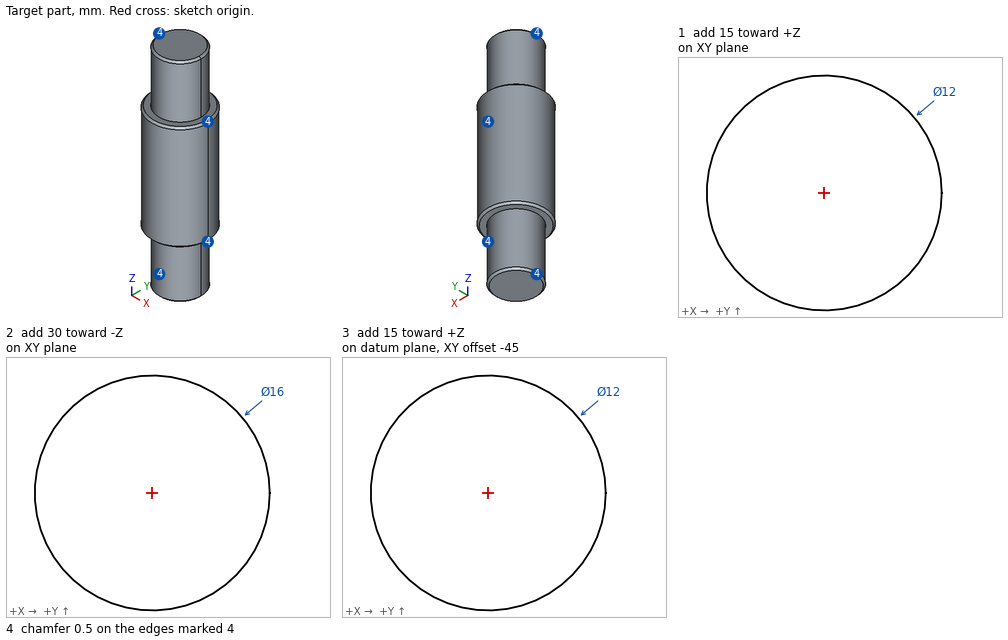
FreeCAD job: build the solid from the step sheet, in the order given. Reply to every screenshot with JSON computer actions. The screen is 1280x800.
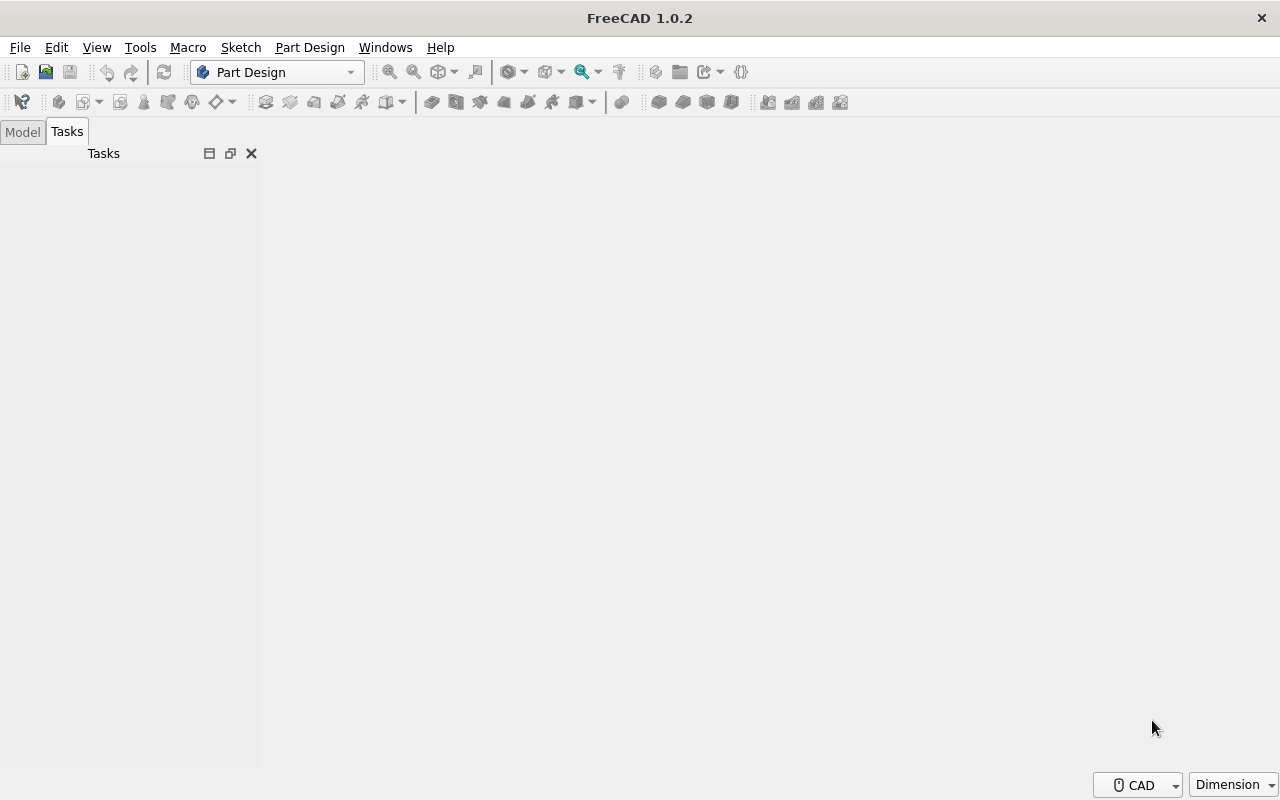
{"action": "left_click", "coordinate": [22, 72]}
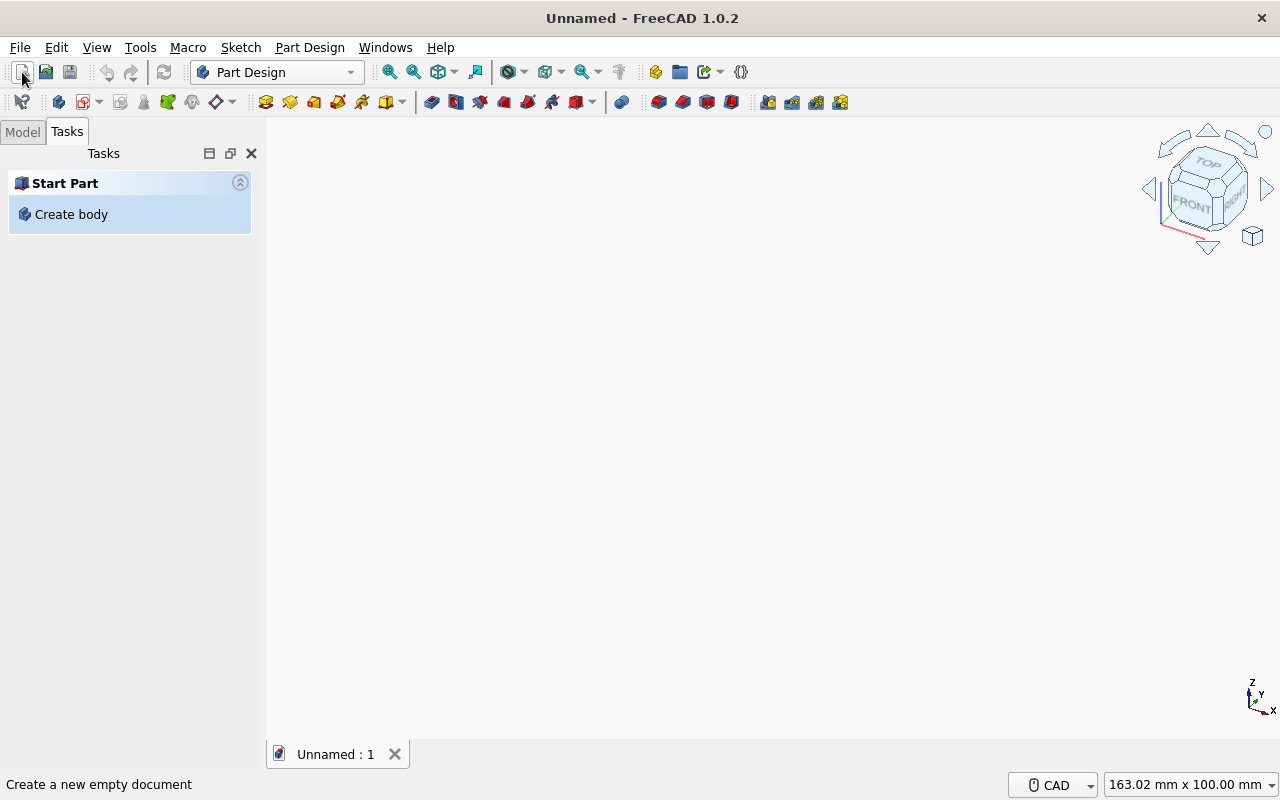
{"action": "left_click", "coordinate": [84, 102]}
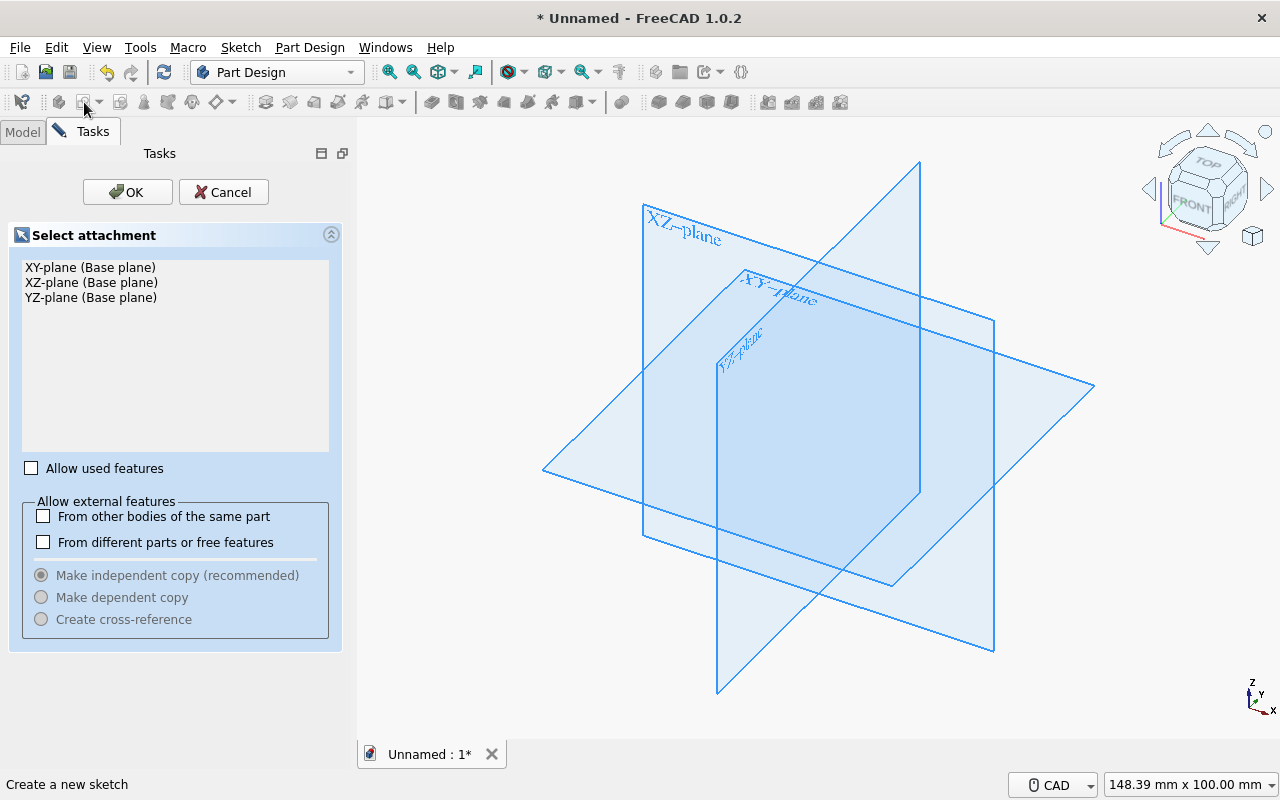
{"action": "left_click", "coordinate": [82, 268]}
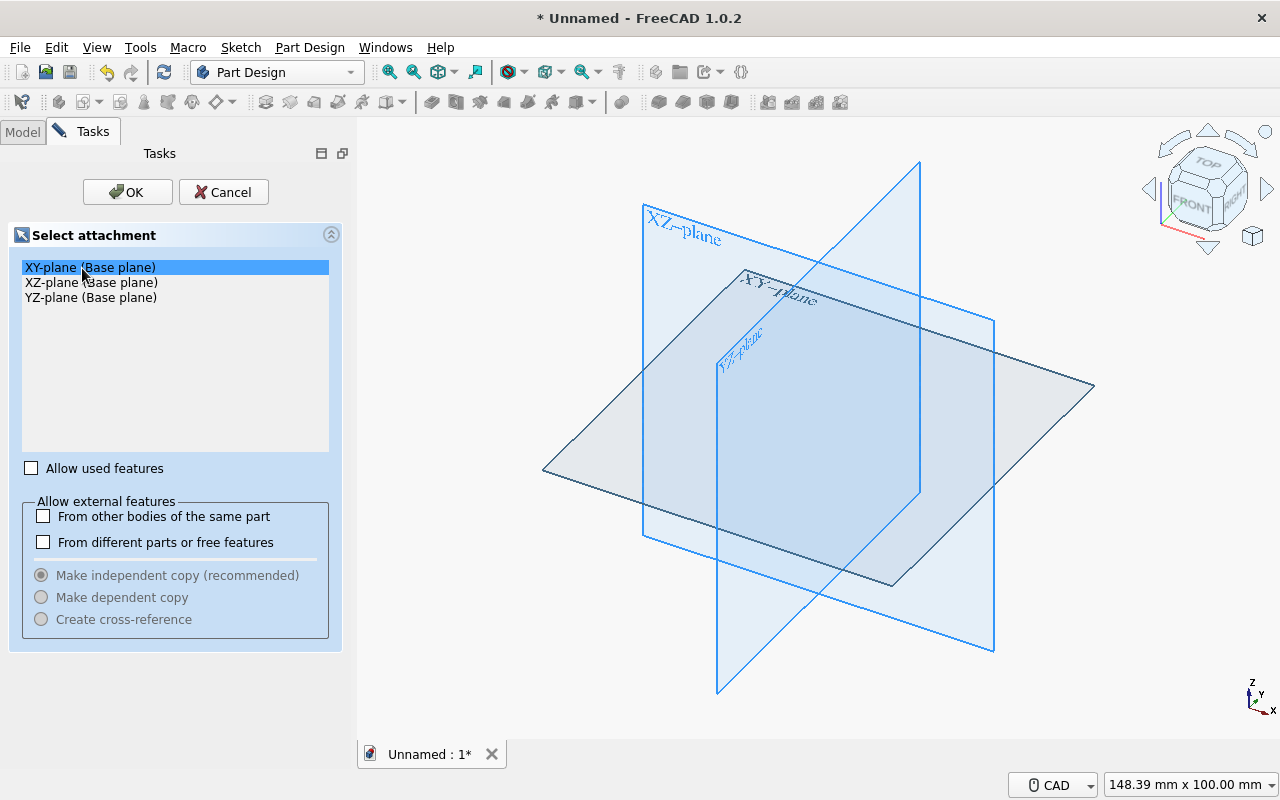
{"action": "left_click", "coordinate": [128, 192]}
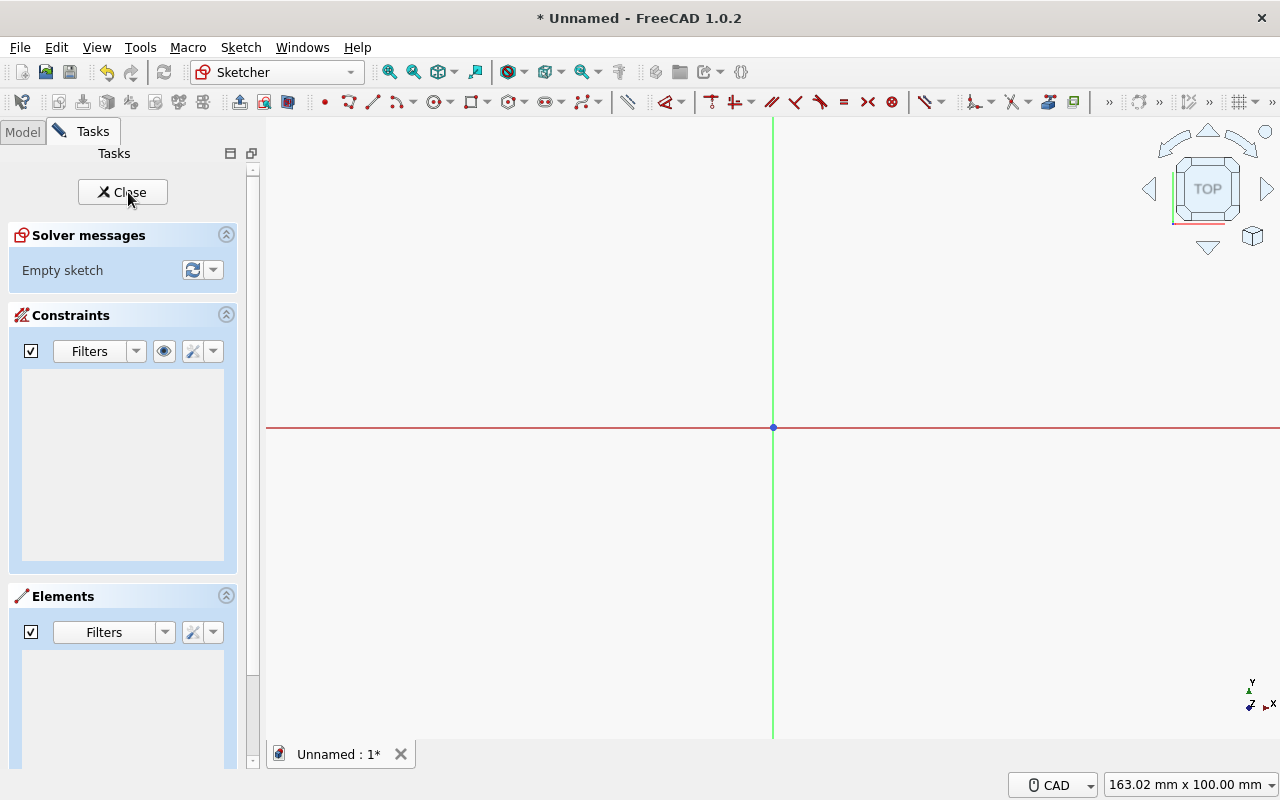
{"action": "scroll", "coordinate": [790, 428], "scroll_direction": "up", "scroll_amount": 8}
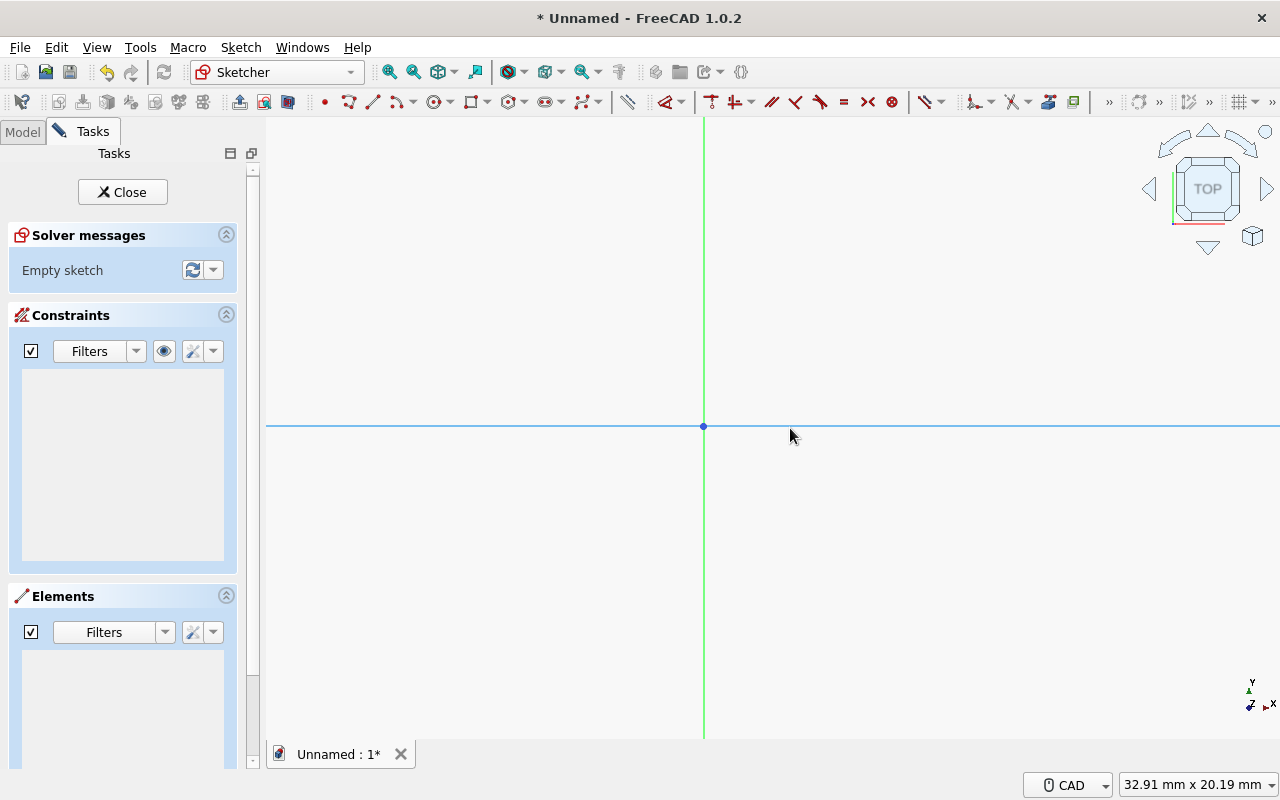
{"action": "left_click", "coordinate": [434, 102]}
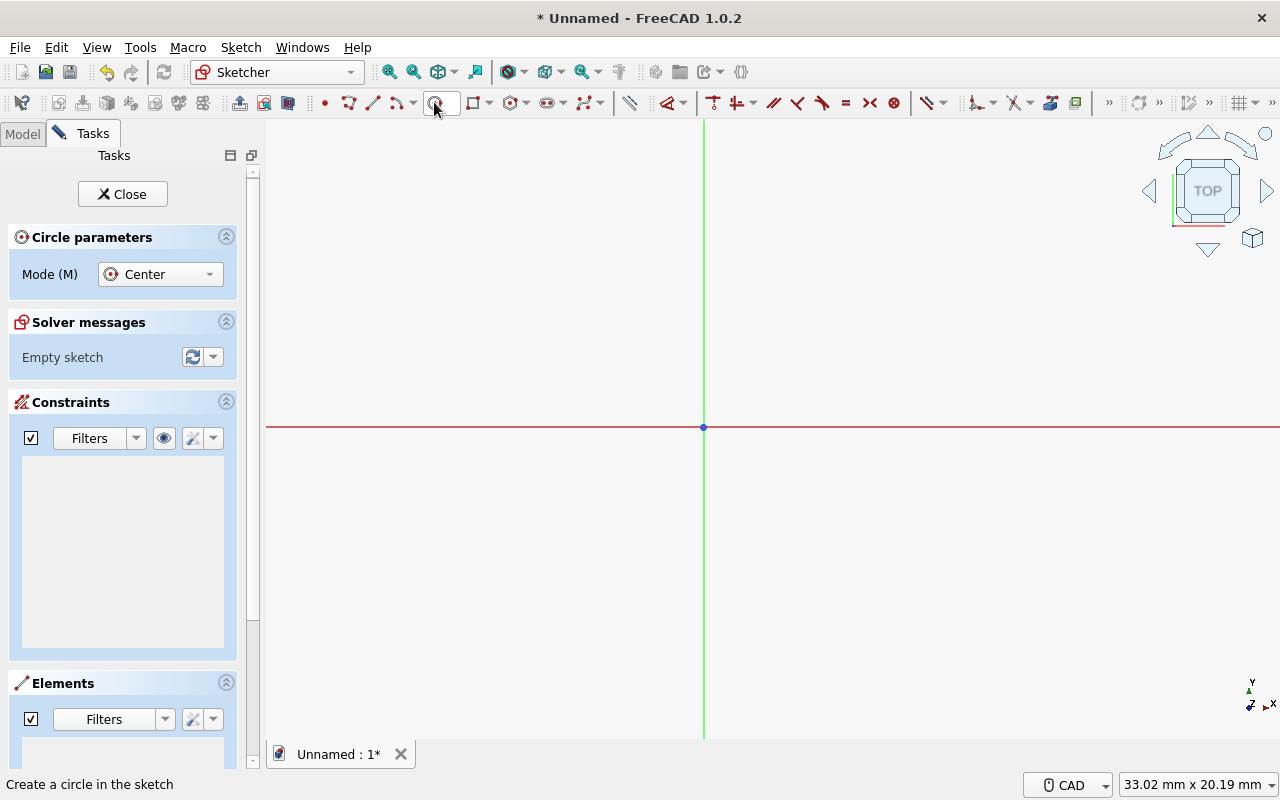
{"action": "left_click", "coordinate": [704, 427]}
{"action": "left_click", "coordinate": [834, 297]}
{"action": "key", "text": "Escape"}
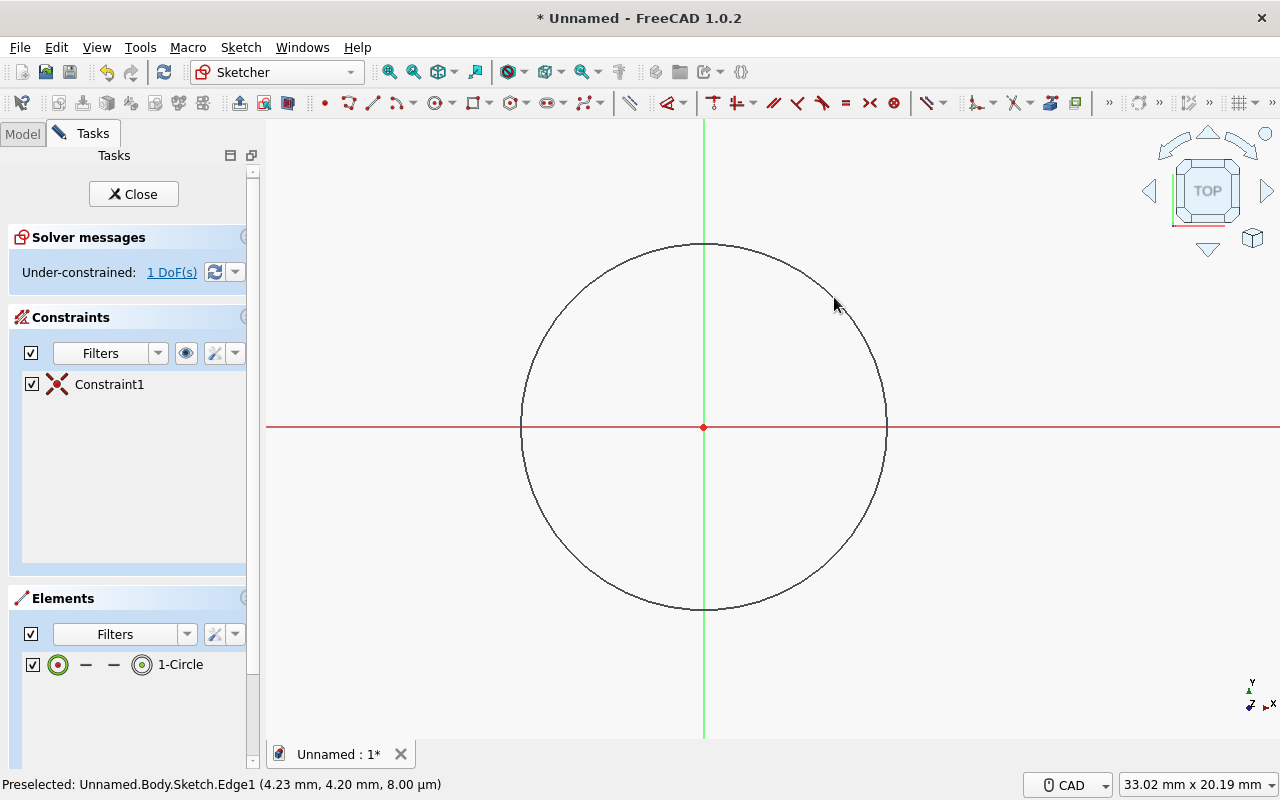
{"action": "left_click", "coordinate": [668, 104]}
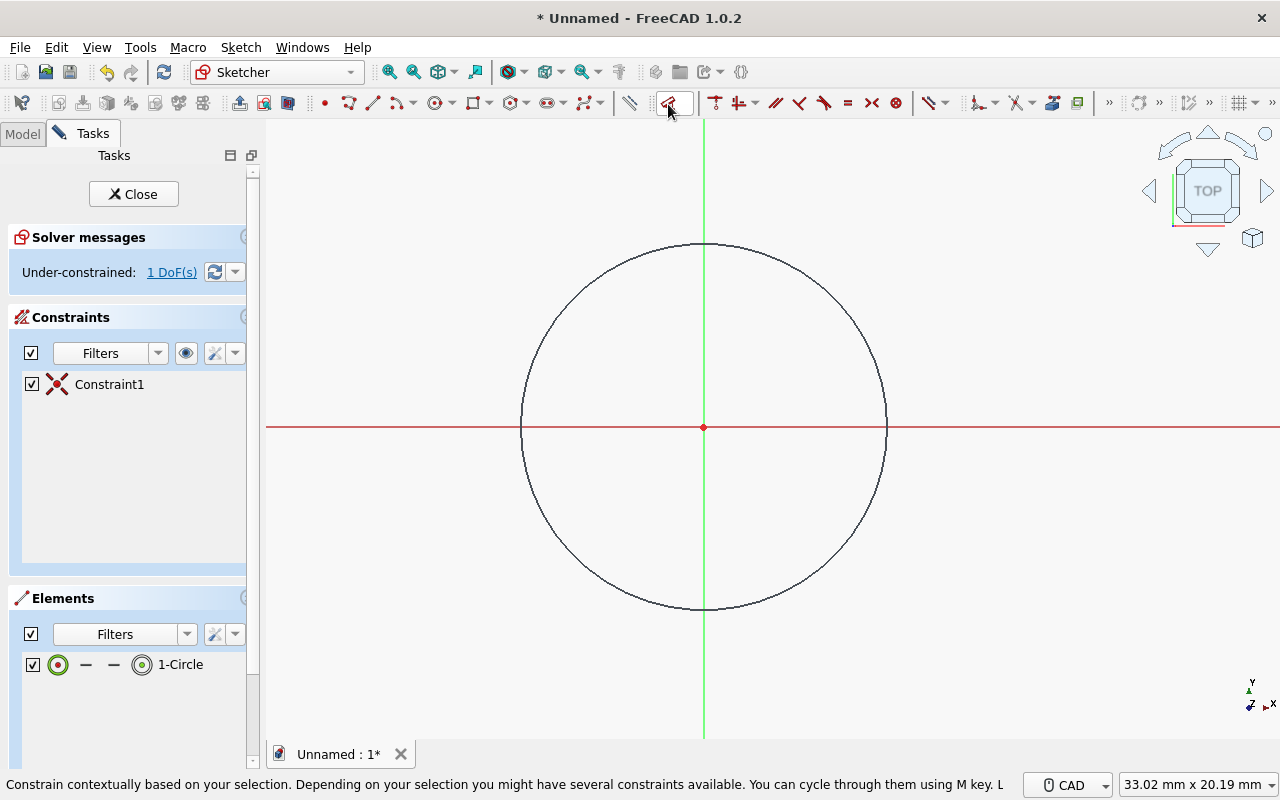
{"action": "left_click", "coordinate": [833, 297]}
{"action": "left_click", "coordinate": [856, 274]}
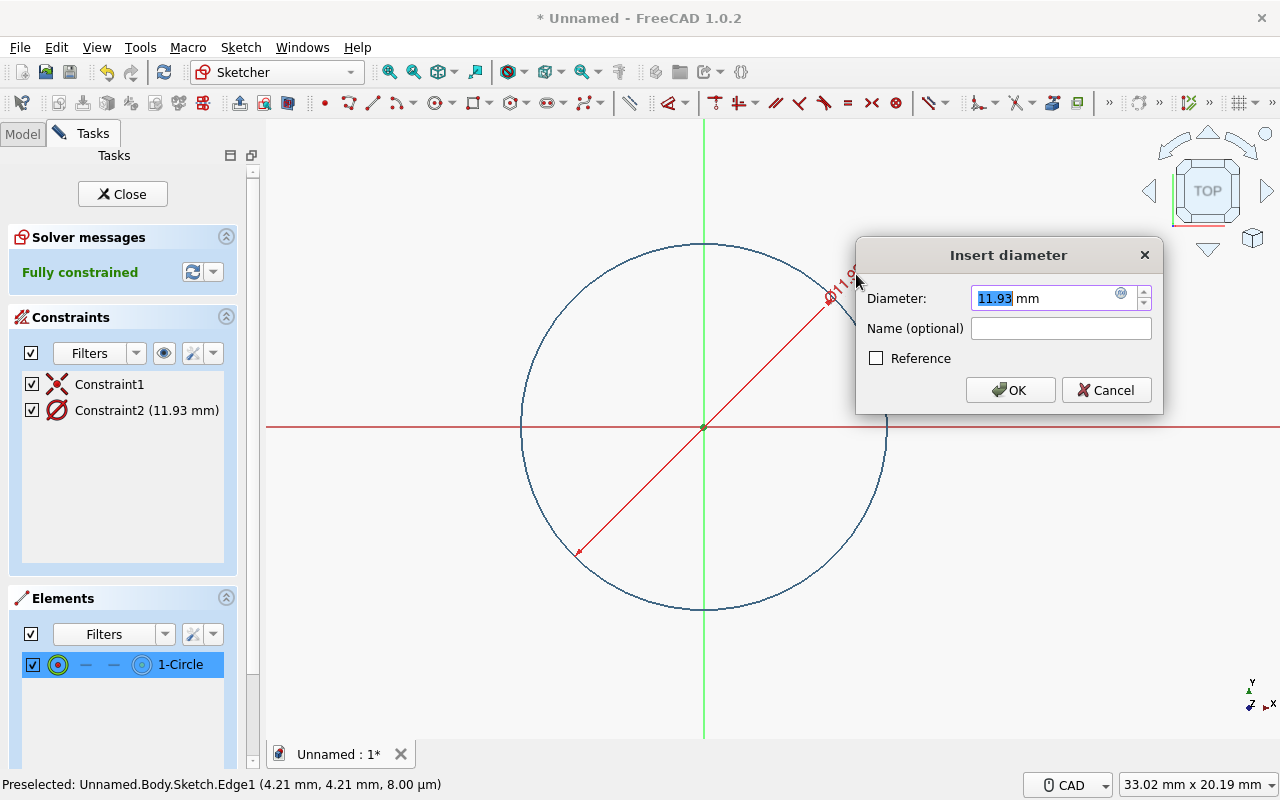
{"action": "type", "text": "12"}
{"action": "key", "text": "Return"}
{"action": "key", "text": "Escape"}